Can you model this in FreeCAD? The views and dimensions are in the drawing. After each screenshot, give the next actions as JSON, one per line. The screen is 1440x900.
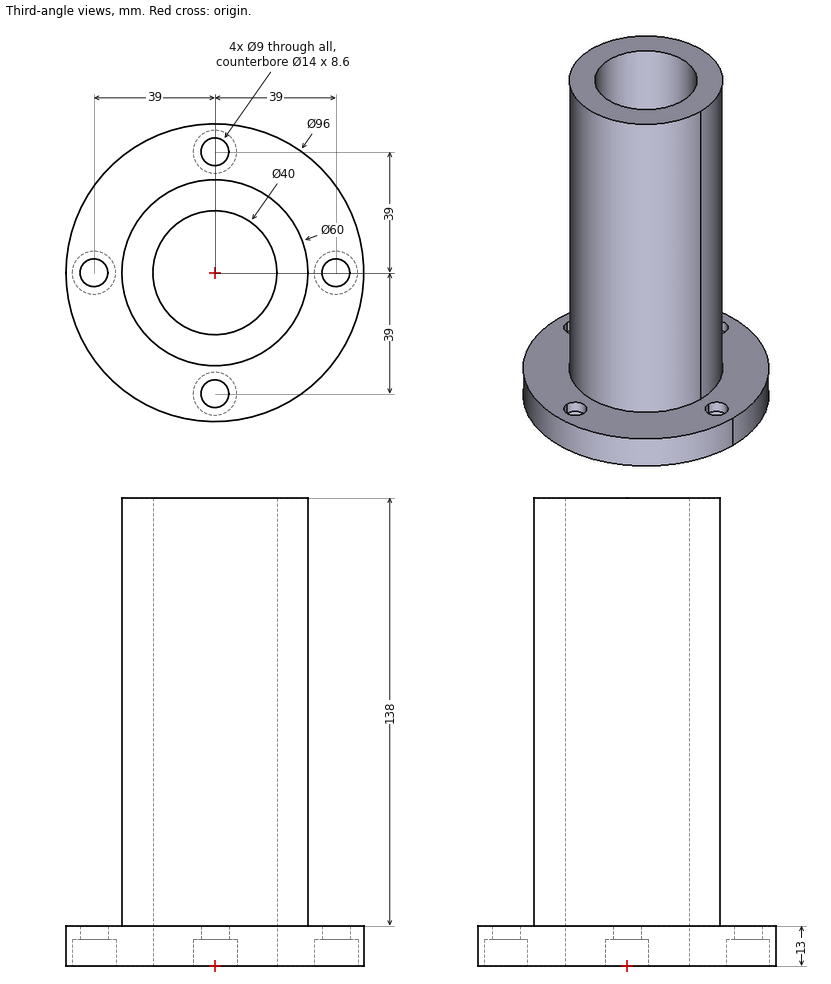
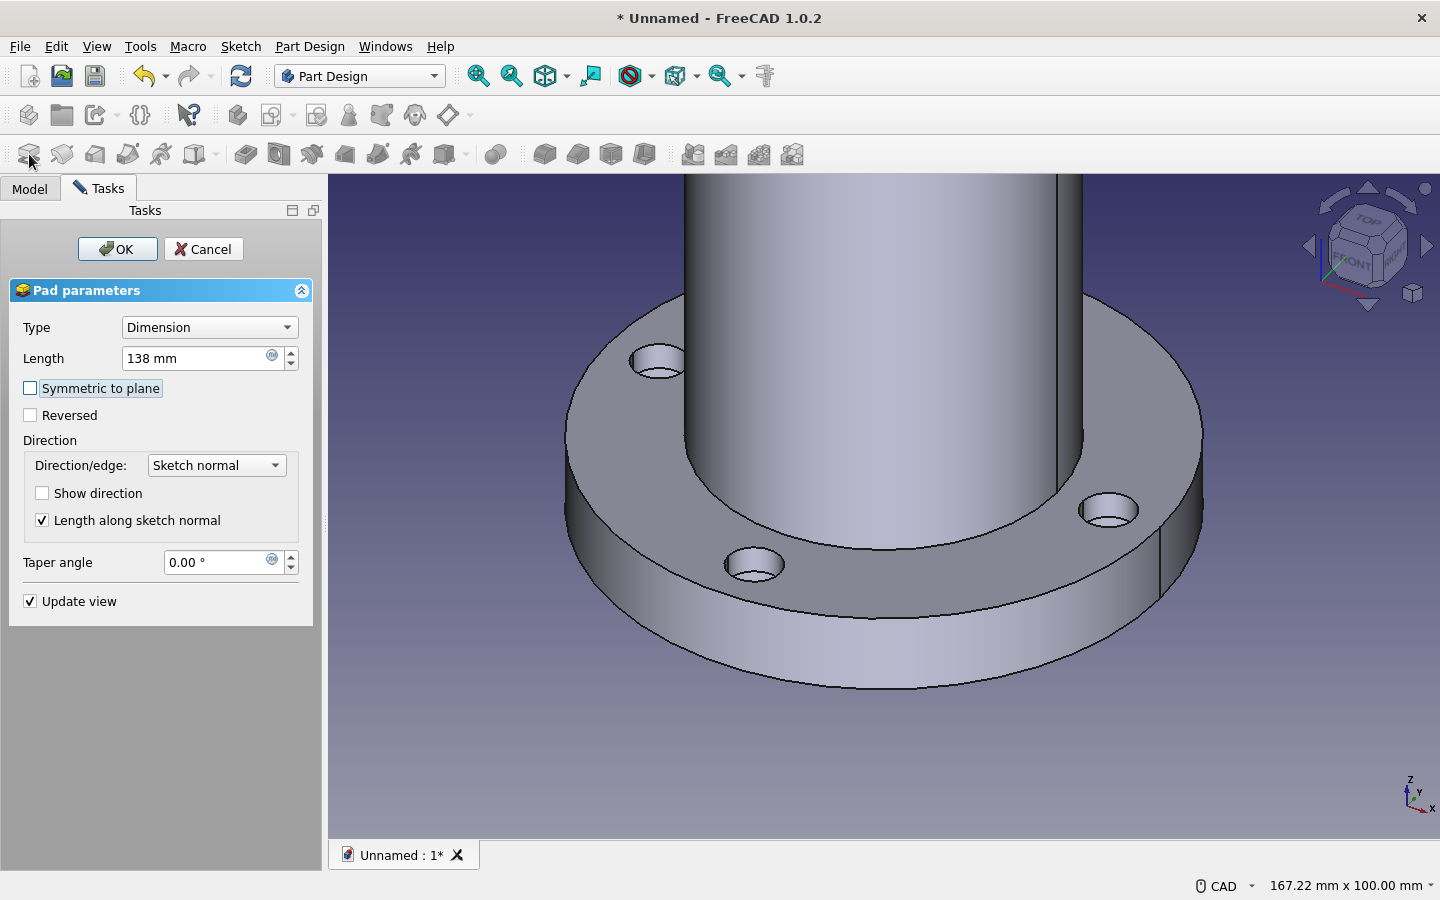
{"action": "left_click", "coordinate": [118, 249]}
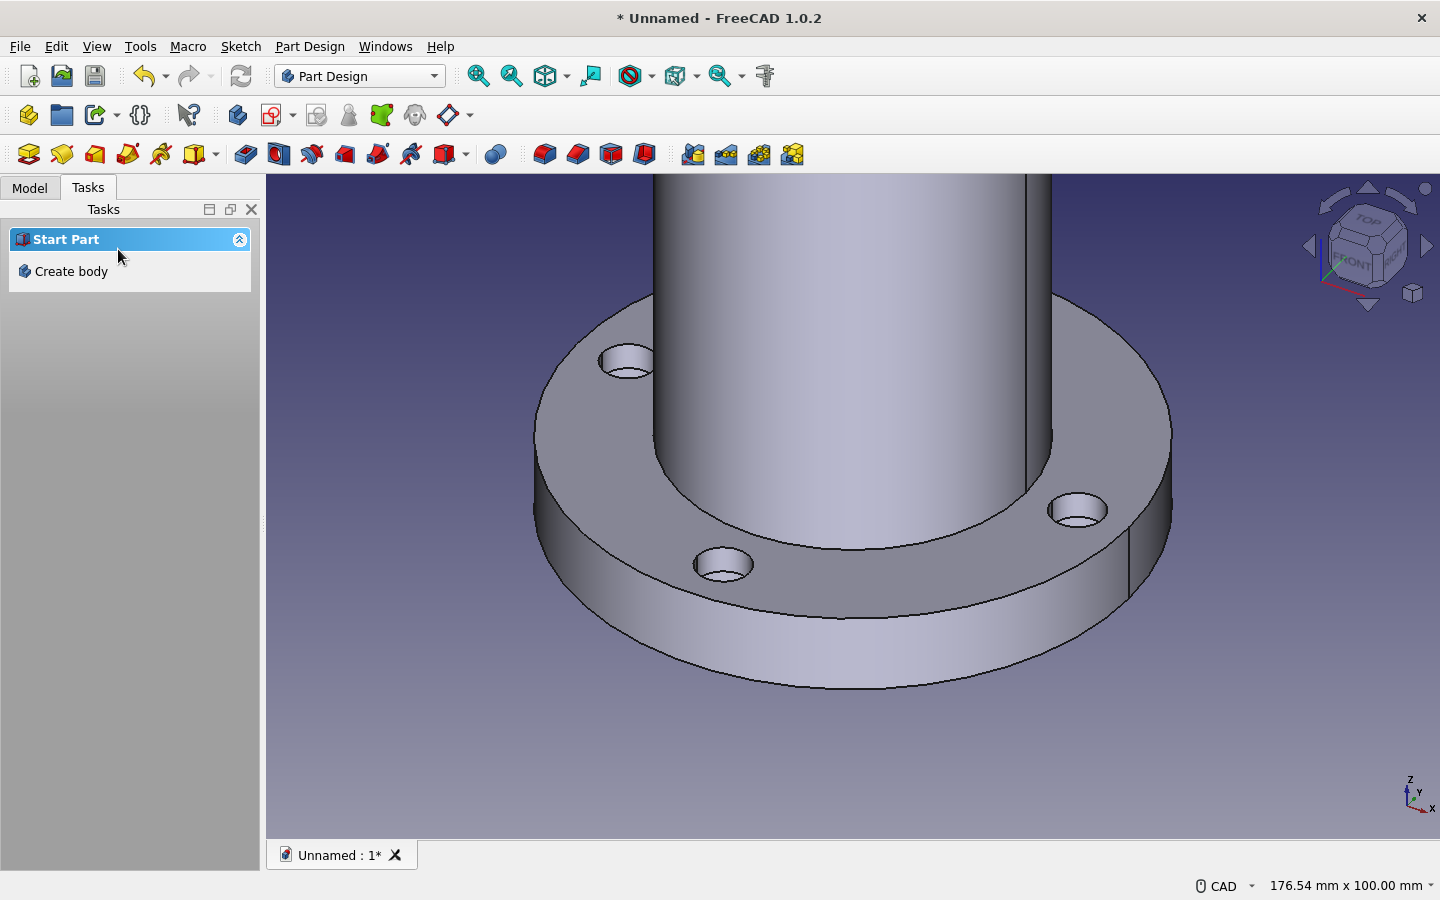
{"action": "left_click", "coordinate": [479, 76]}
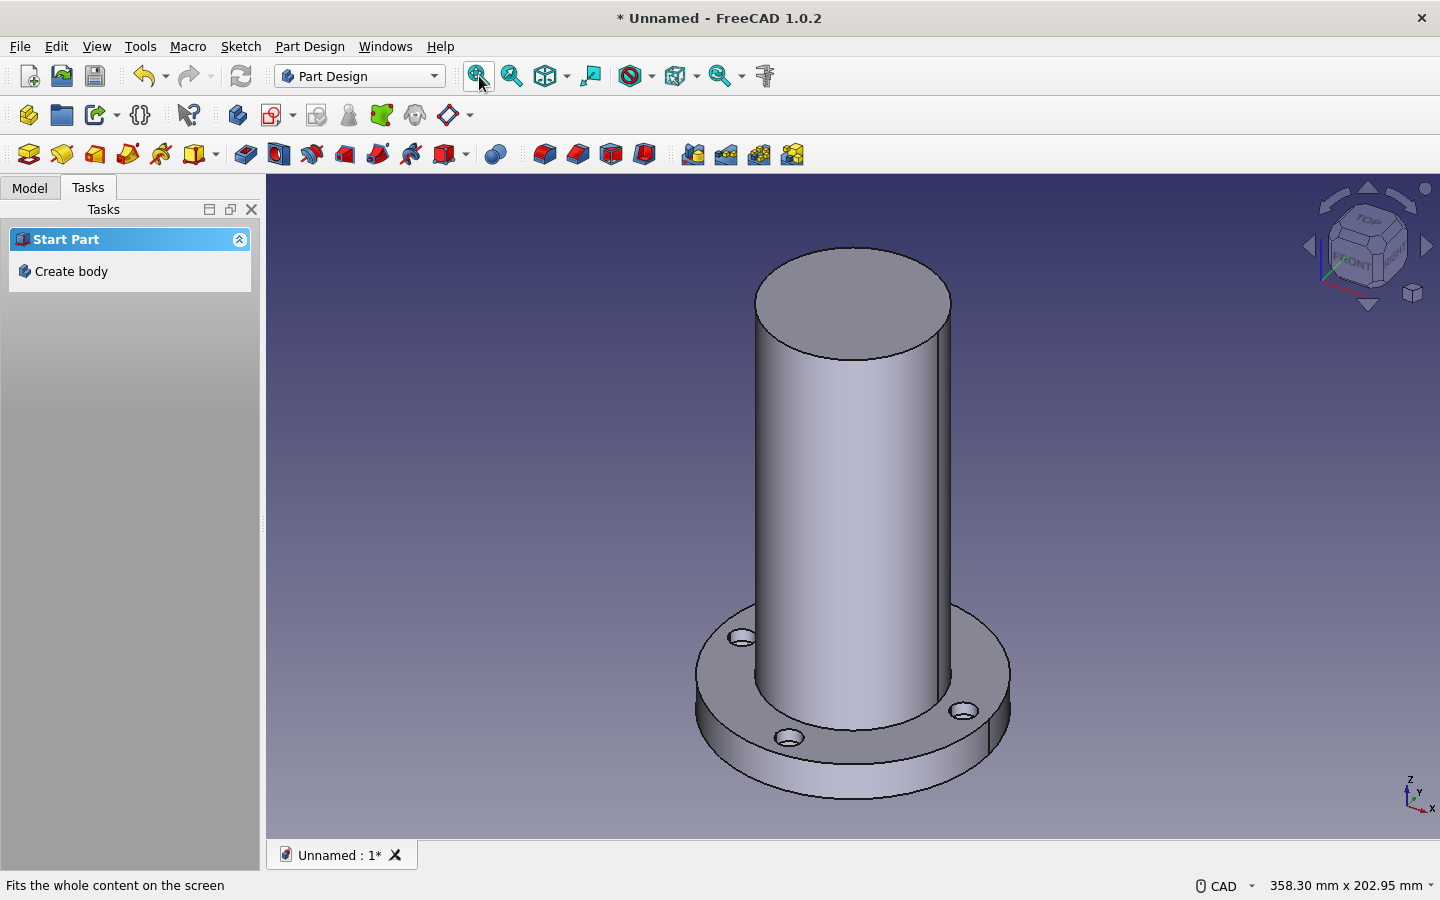
{"action": "left_click", "coordinate": [853, 303]}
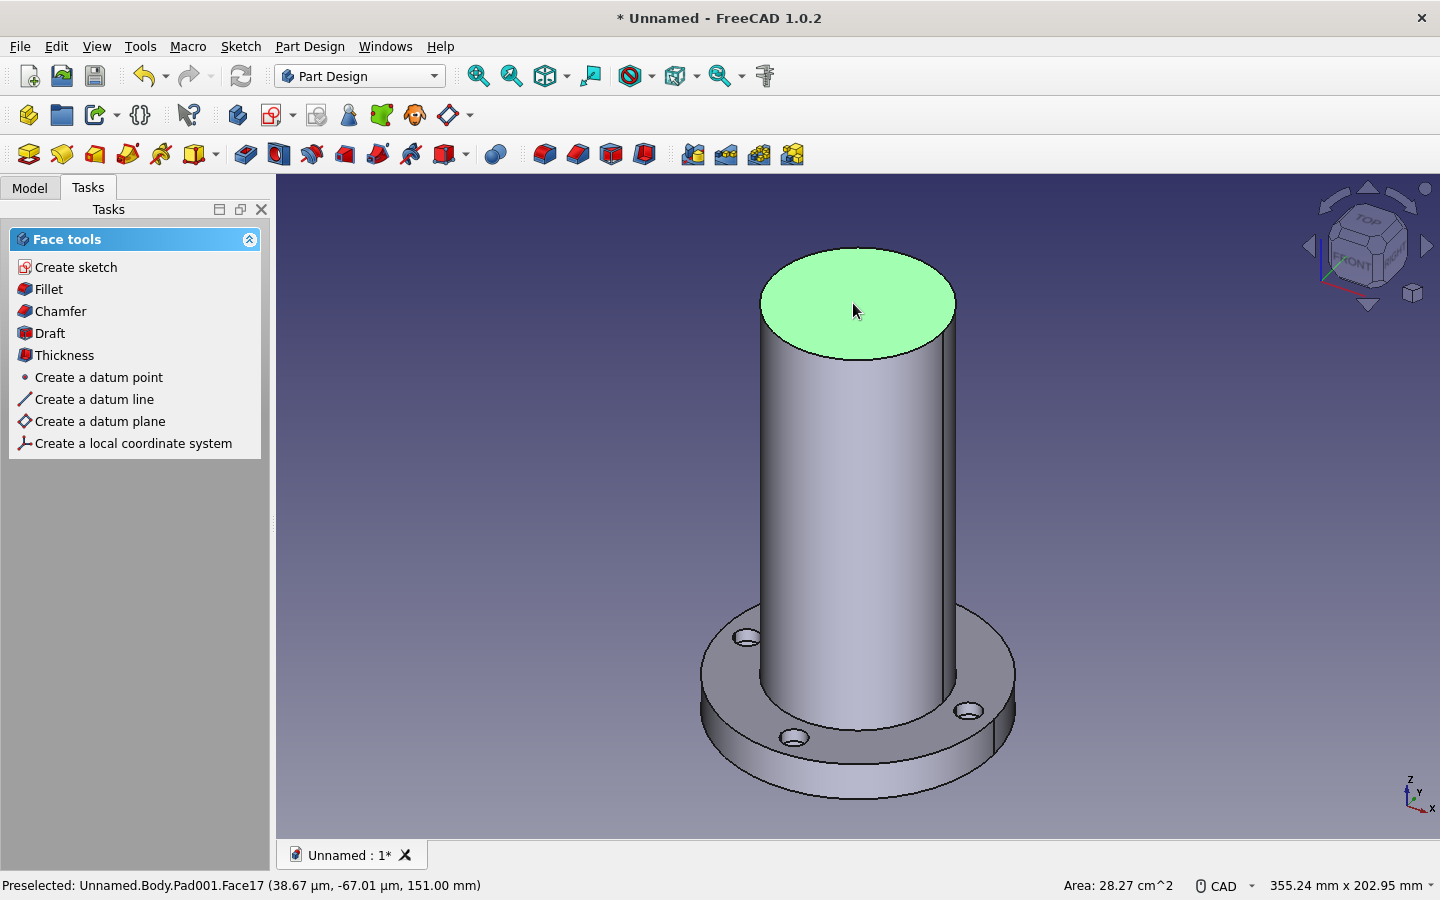
{"action": "left_click", "coordinate": [270, 116]}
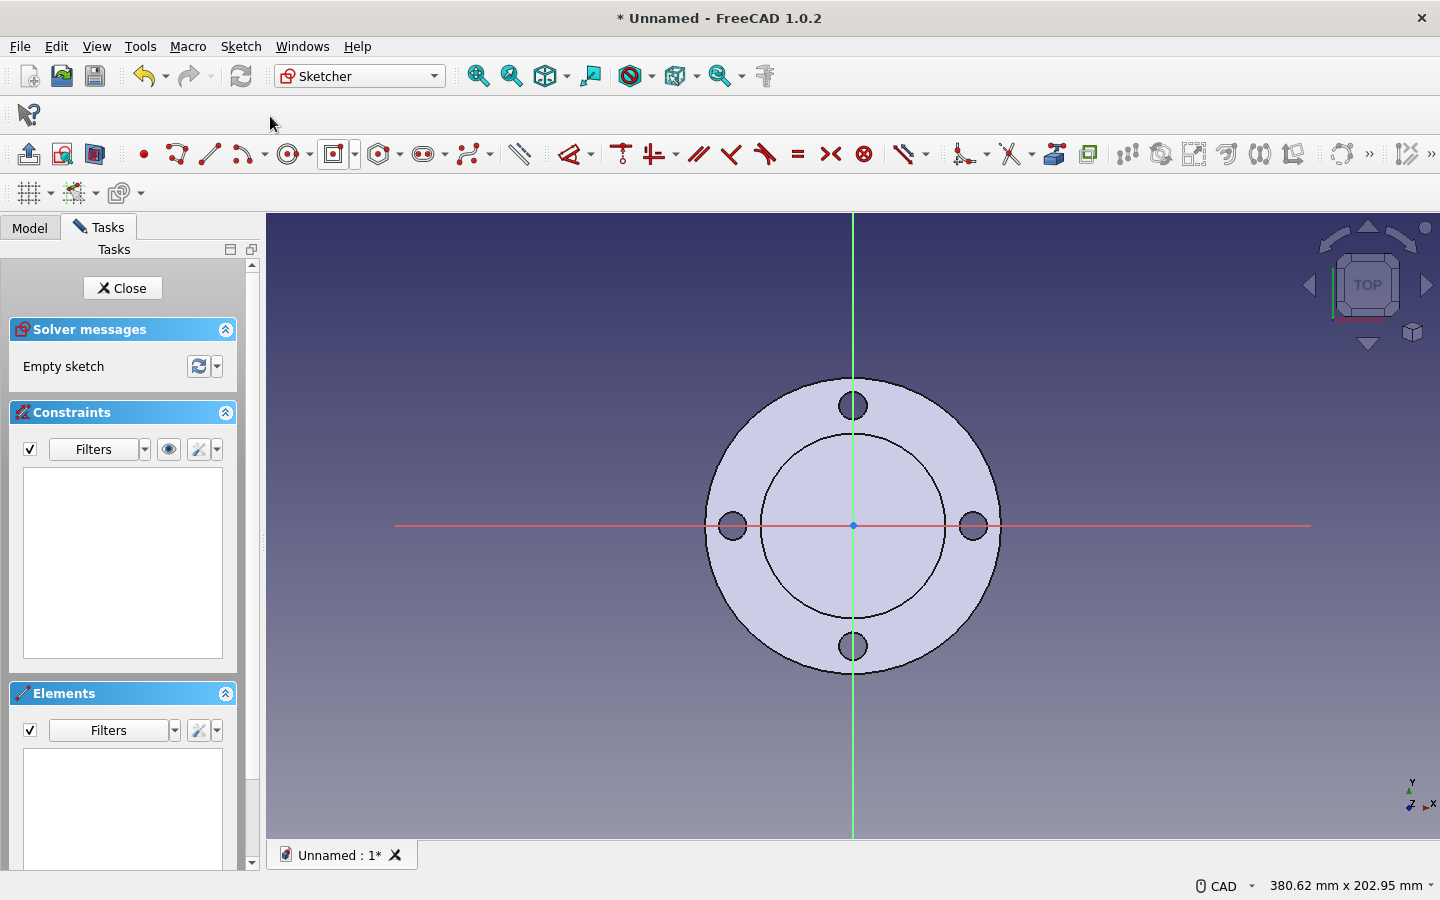
{"action": "scroll", "coordinate": [883, 526], "scroll_direction": "up", "scroll_amount": 6}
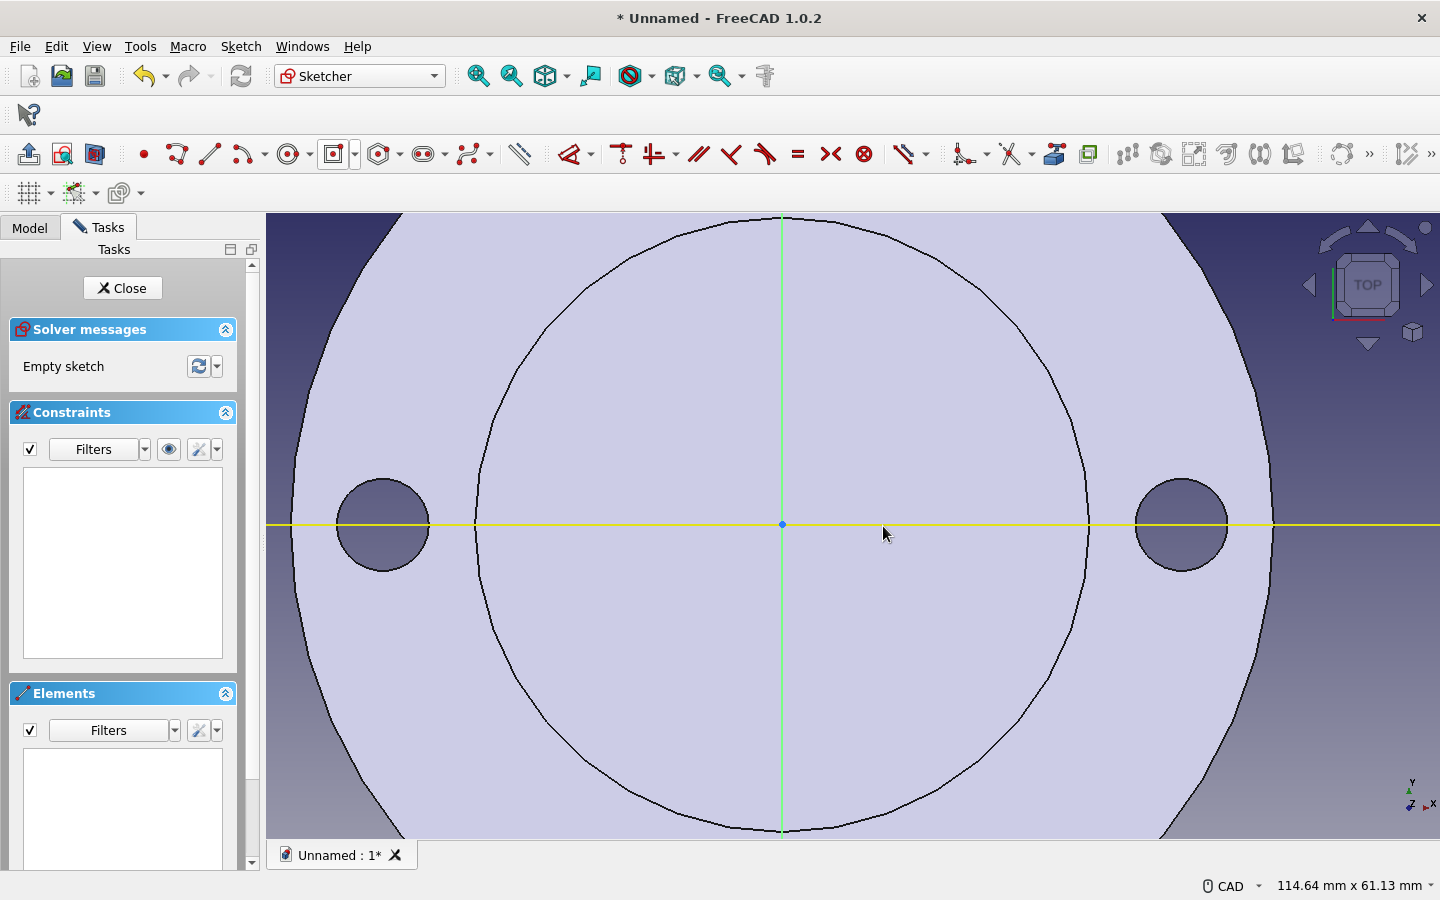
{"action": "left_click", "coordinate": [288, 154]}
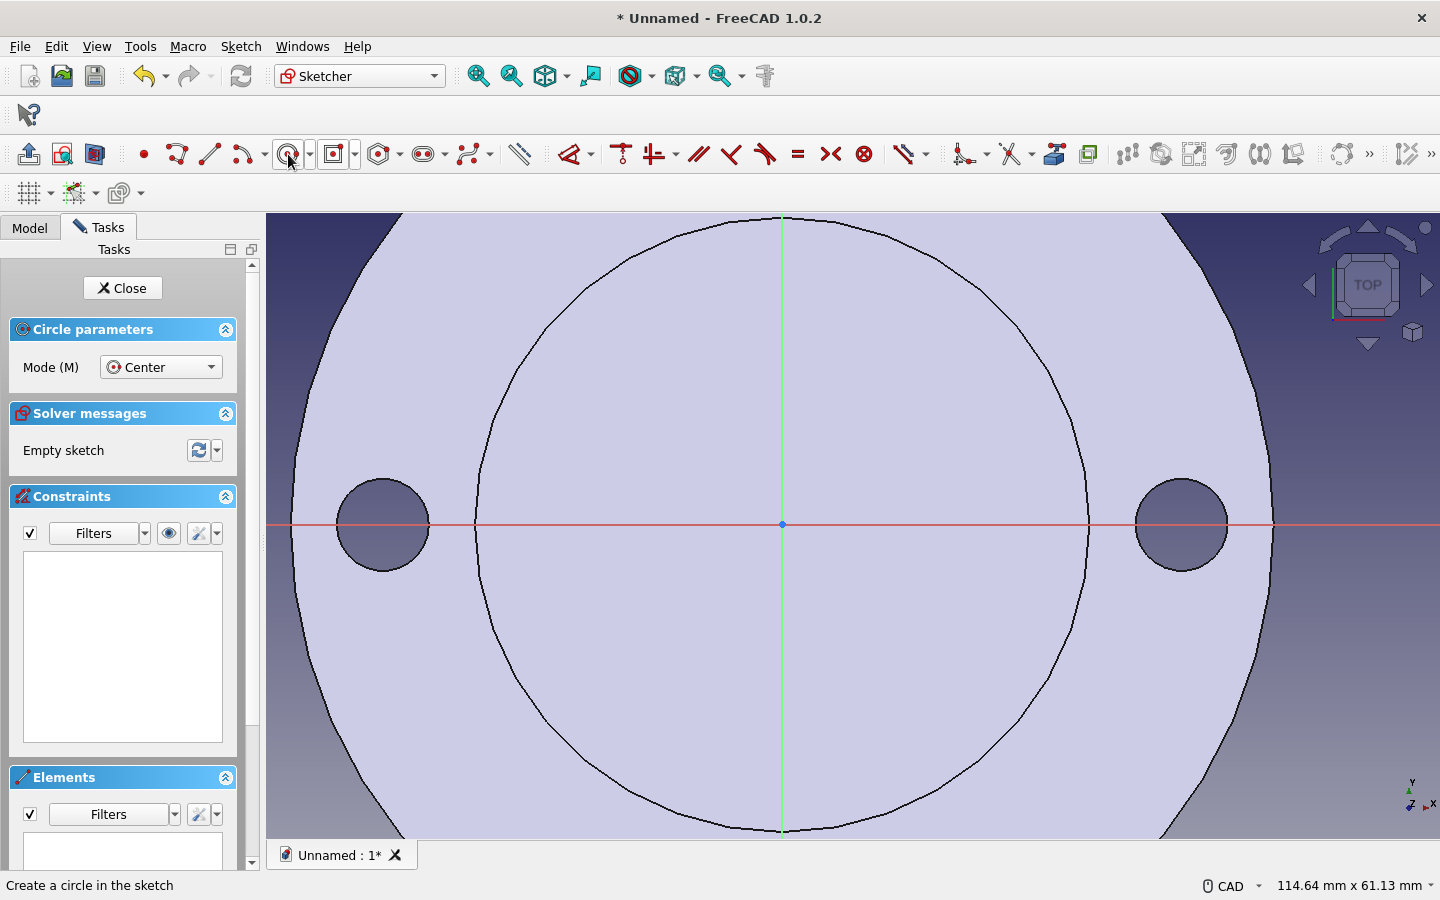
{"action": "left_click", "coordinate": [782, 525]}
{"action": "mouse_move", "coordinate": [927, 380]}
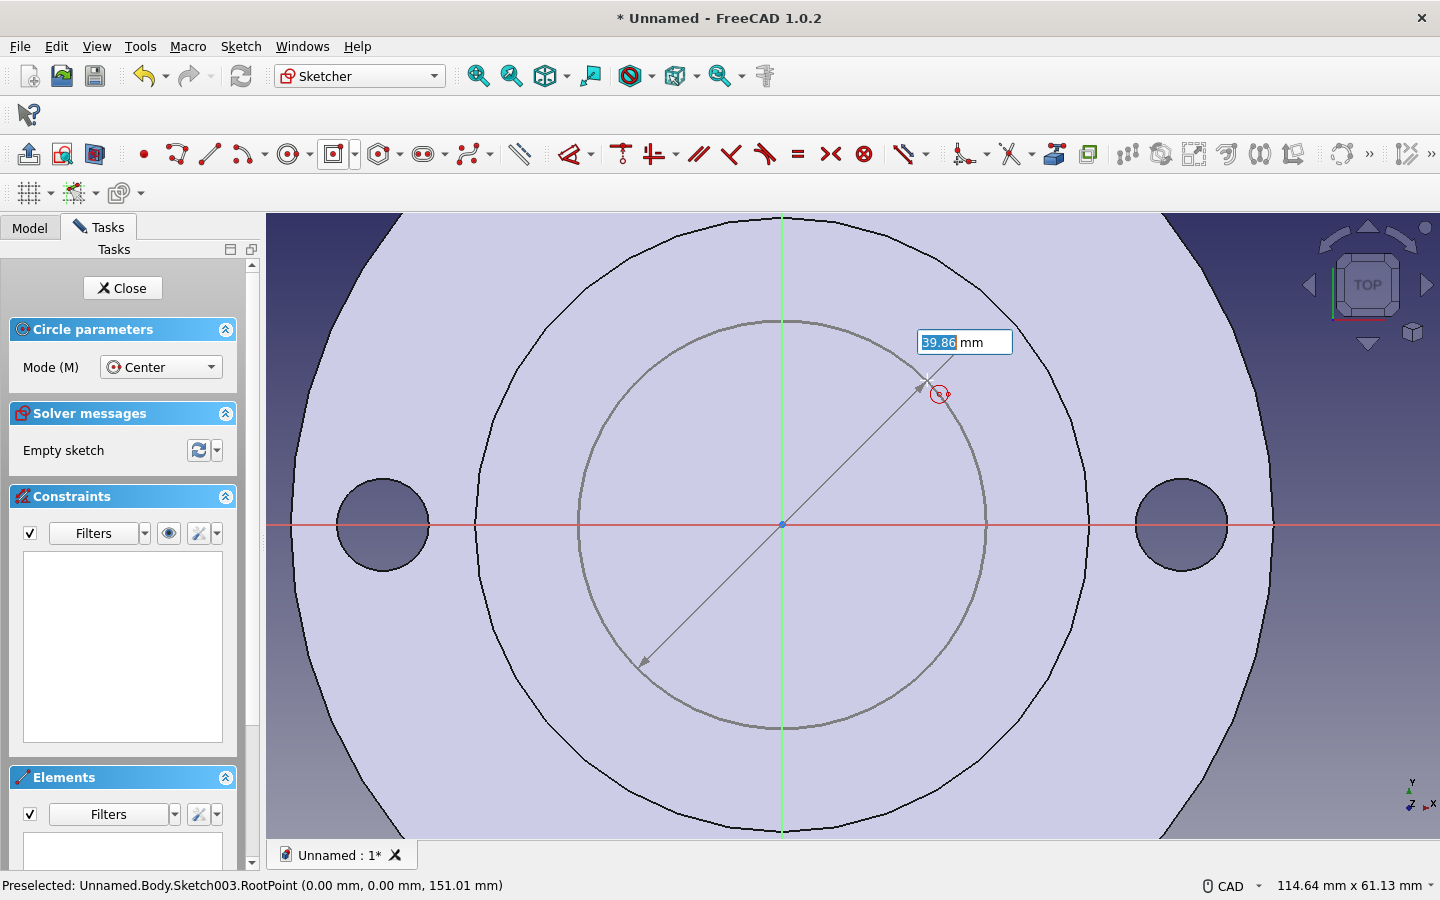
{"action": "type", "text": "40"}
{"action": "key", "text": "Return"}
{"action": "key", "text": "Escape"}